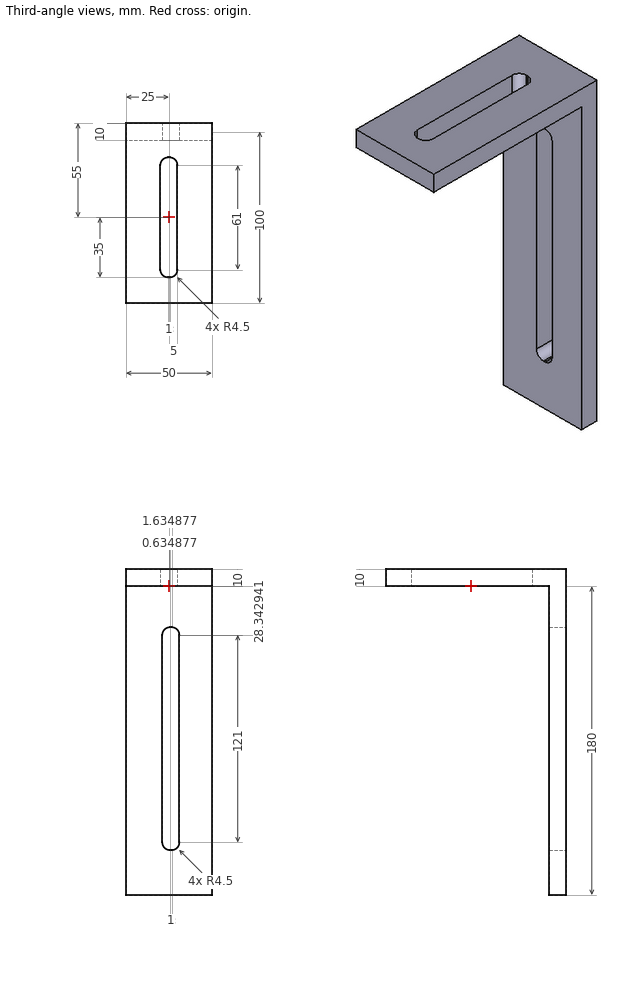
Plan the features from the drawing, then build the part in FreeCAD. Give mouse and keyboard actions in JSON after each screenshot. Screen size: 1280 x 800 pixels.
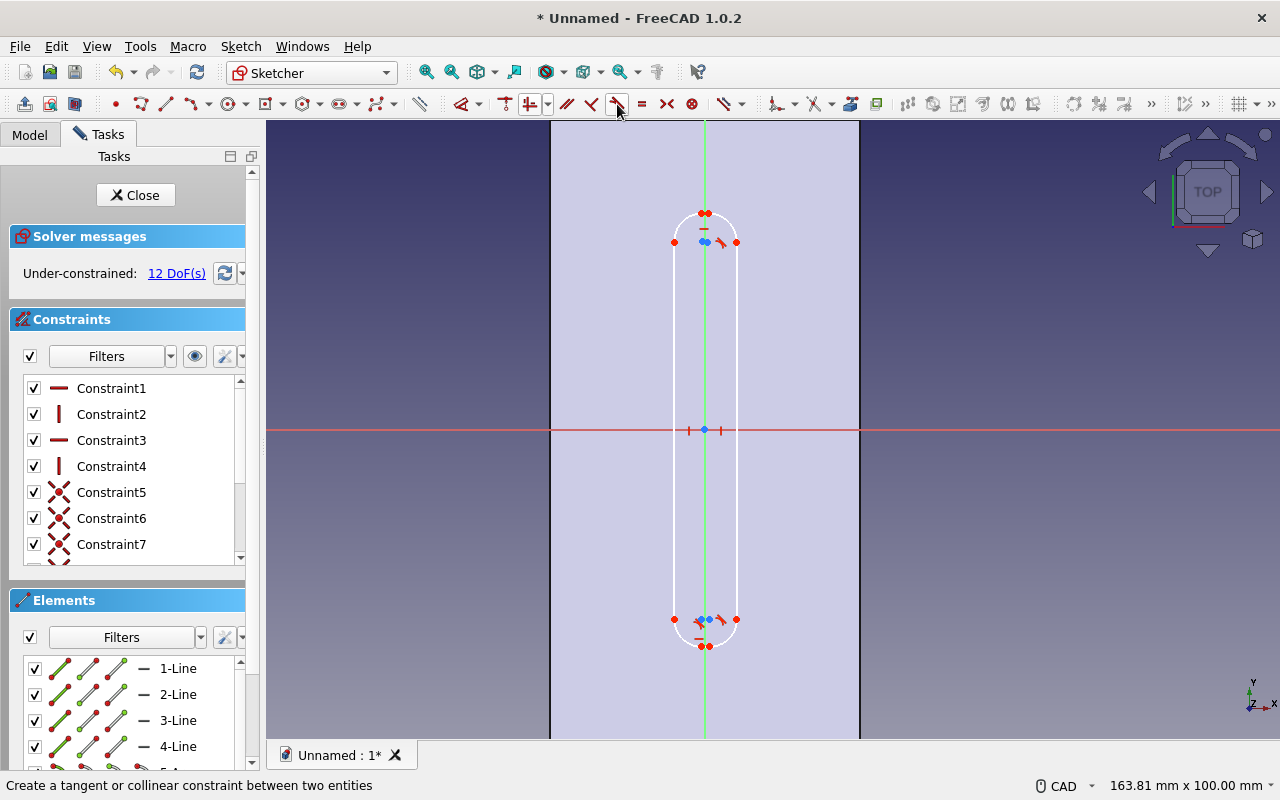
{"action": "scroll", "coordinate": [705, 213], "scroll_direction": "up", "scroll_amount": 8}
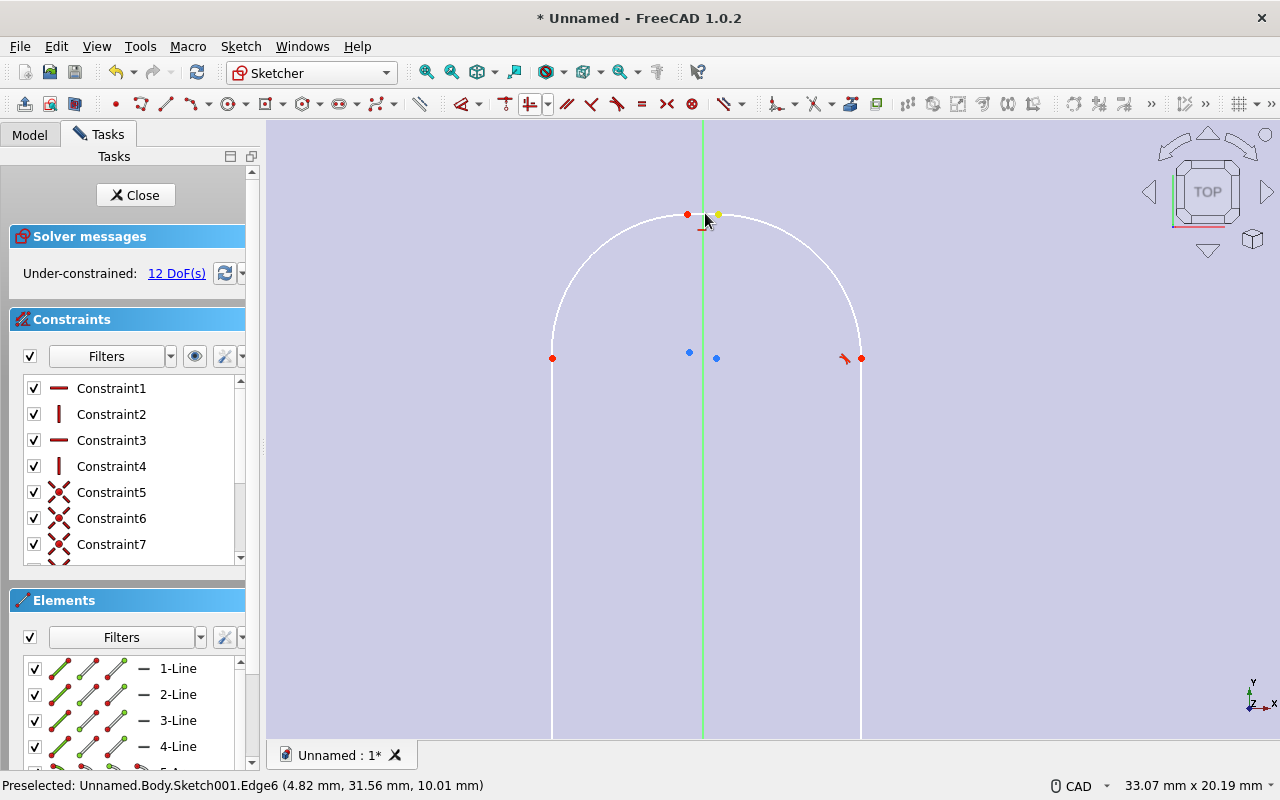
{"action": "left_click", "coordinate": [703, 214]}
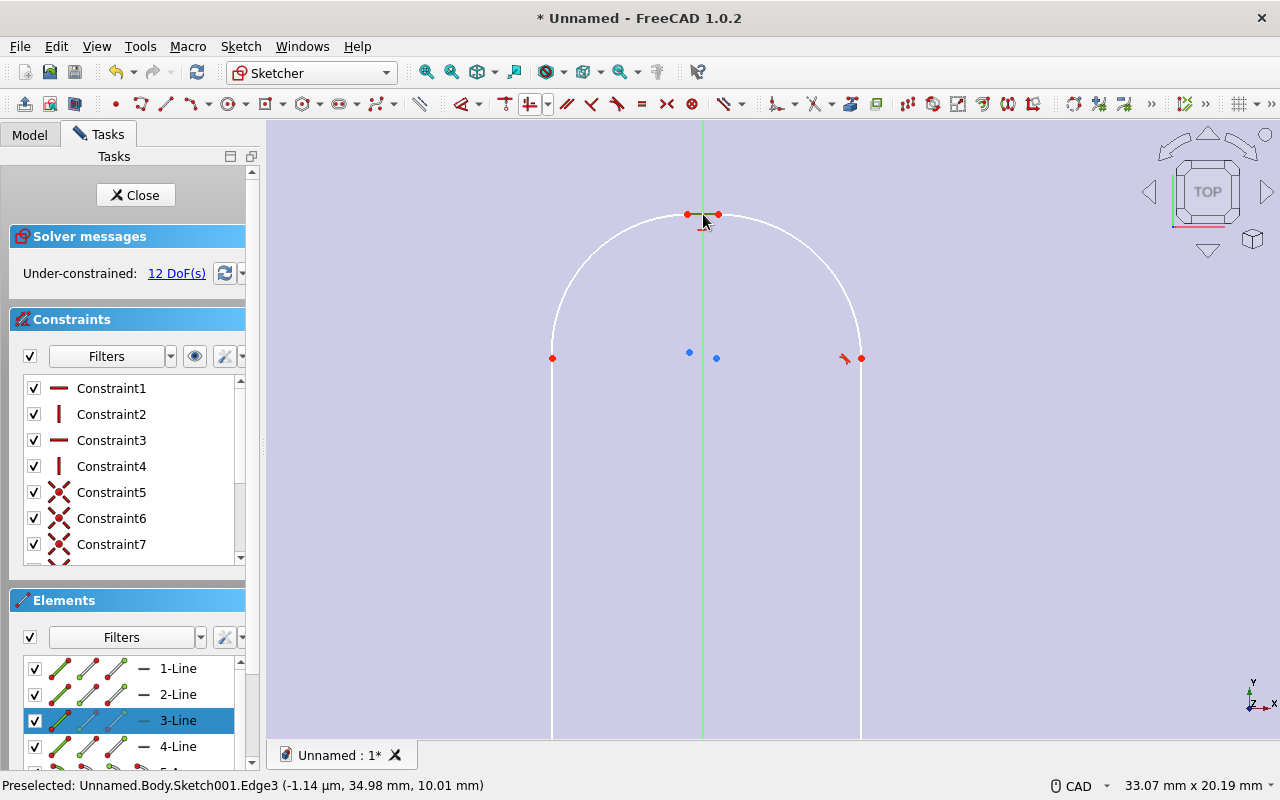
{"action": "scroll", "coordinate": [705, 213], "scroll_direction": "down", "scroll_amount": 8}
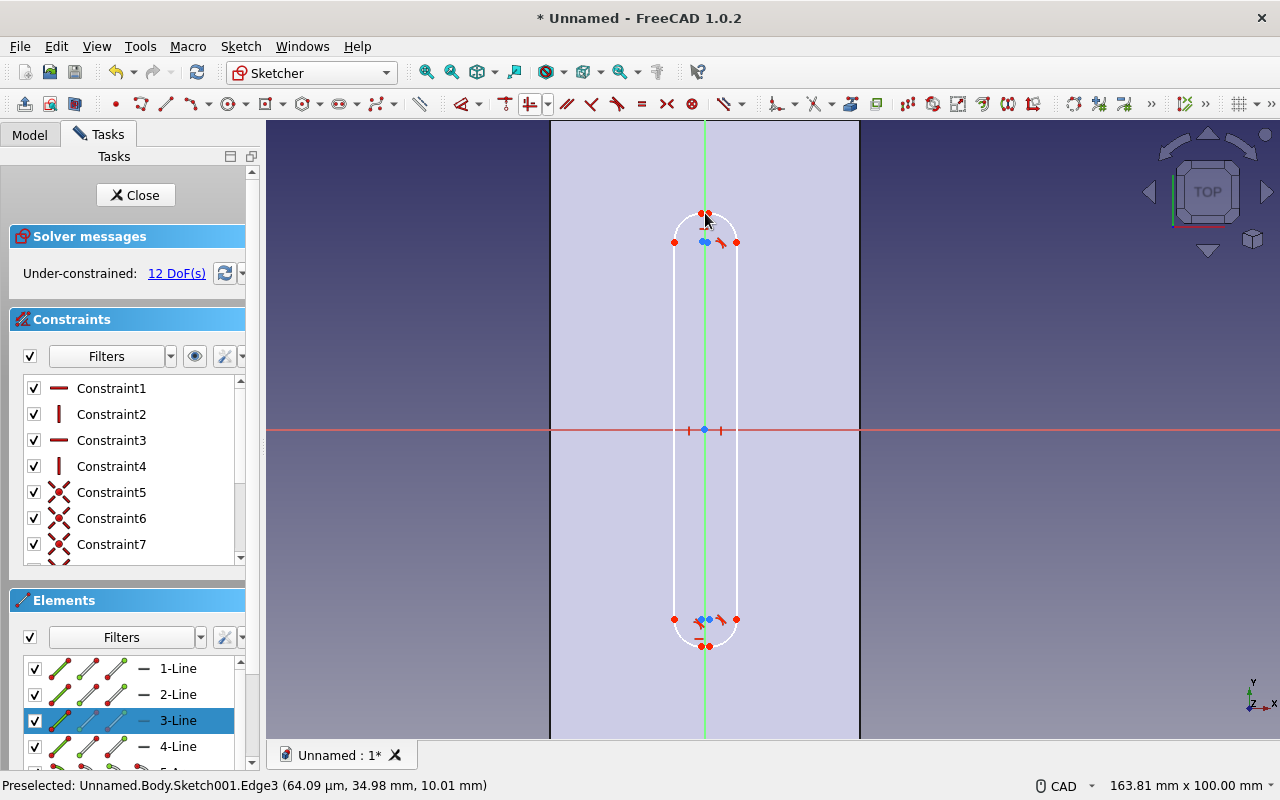
{"action": "left_click", "coordinate": [734, 229]}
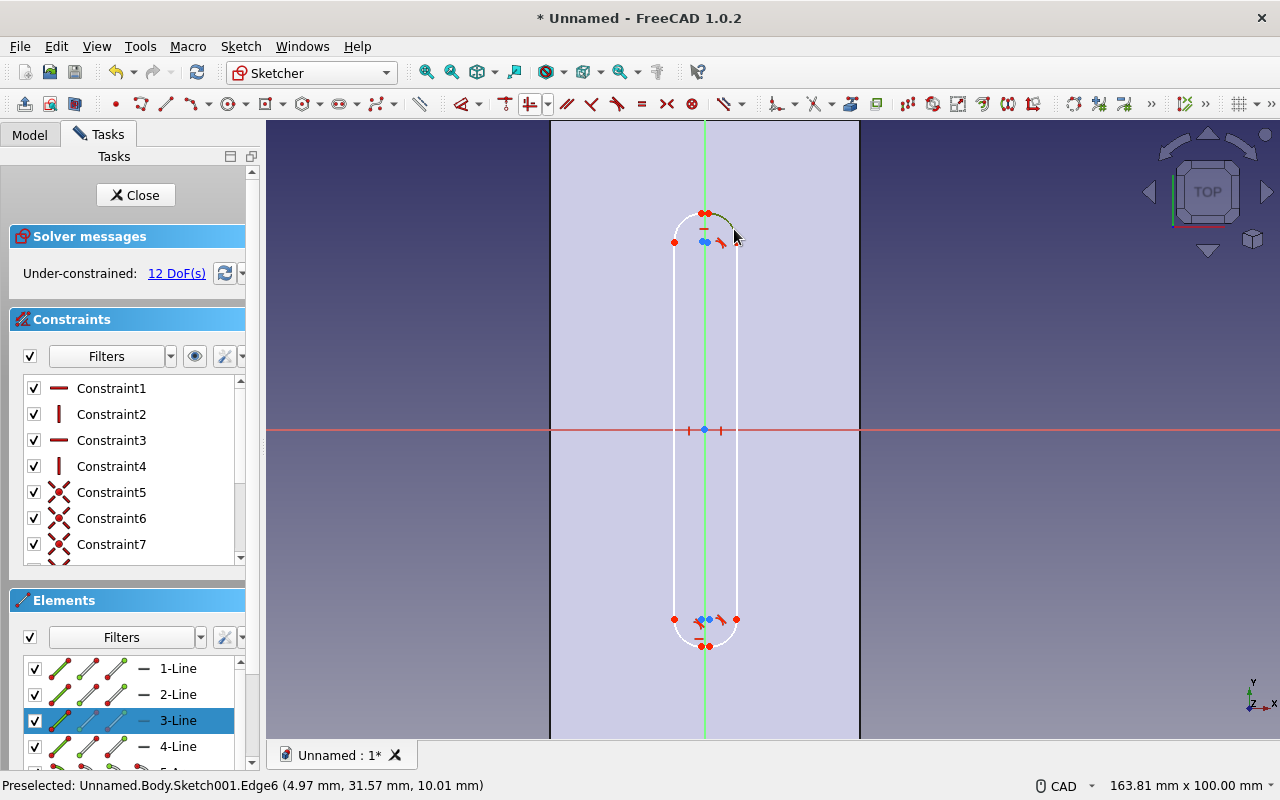
{"action": "left_click", "coordinate": [617, 104]}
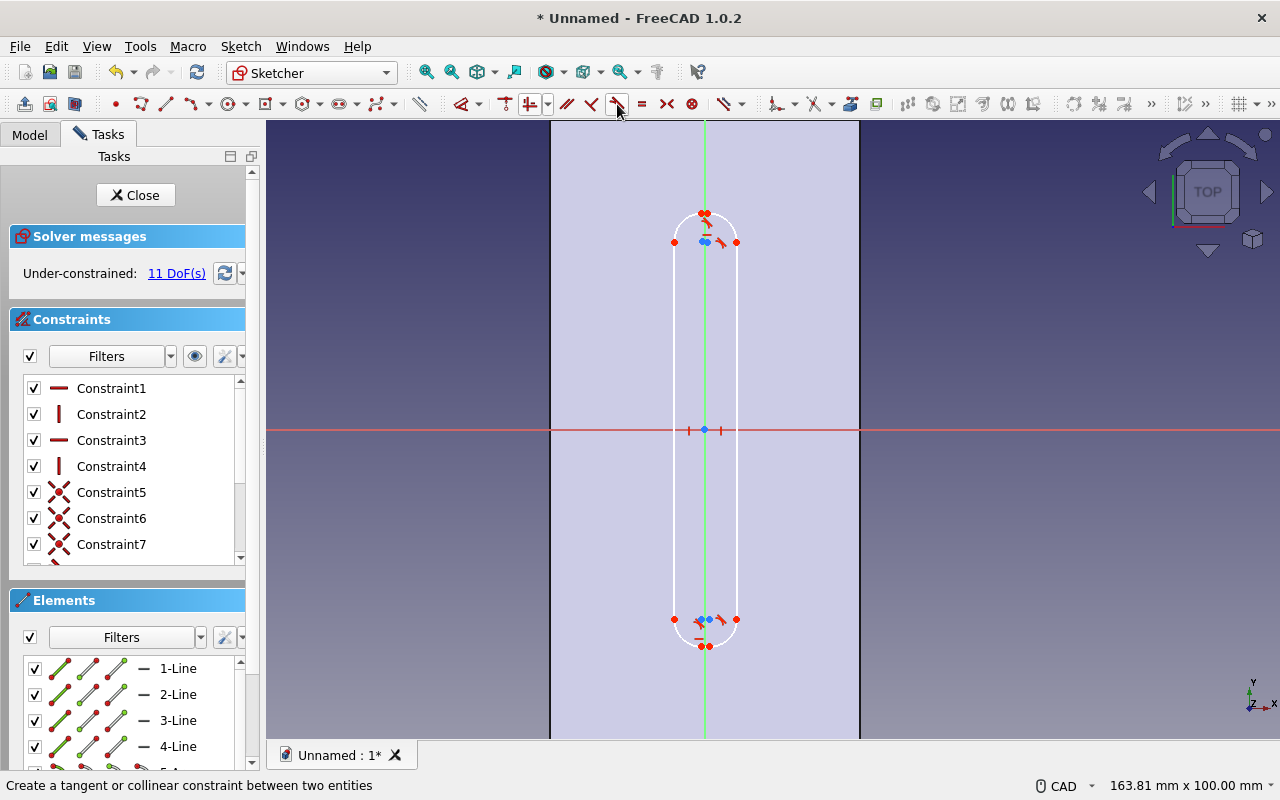
{"action": "scroll", "coordinate": [705, 213], "scroll_direction": "up", "scroll_amount": 8}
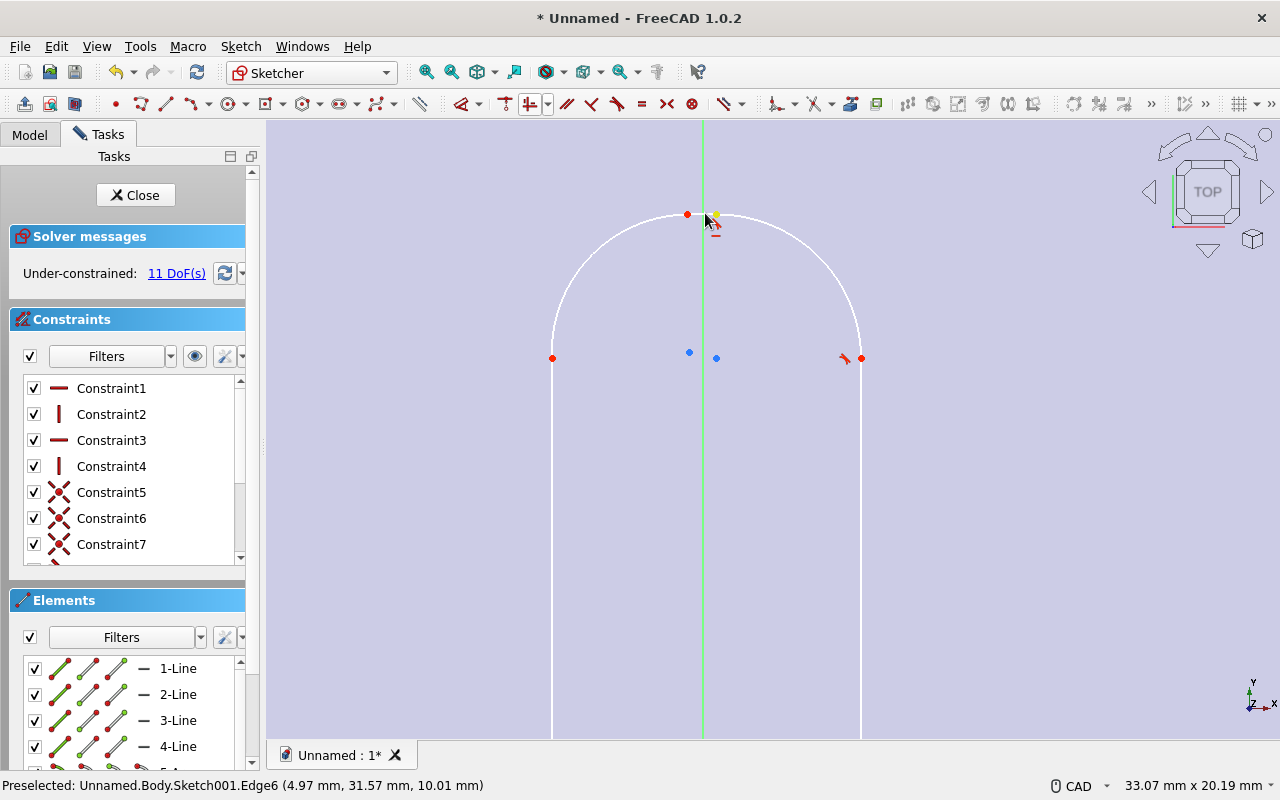
{"action": "left_click", "coordinate": [702, 214]}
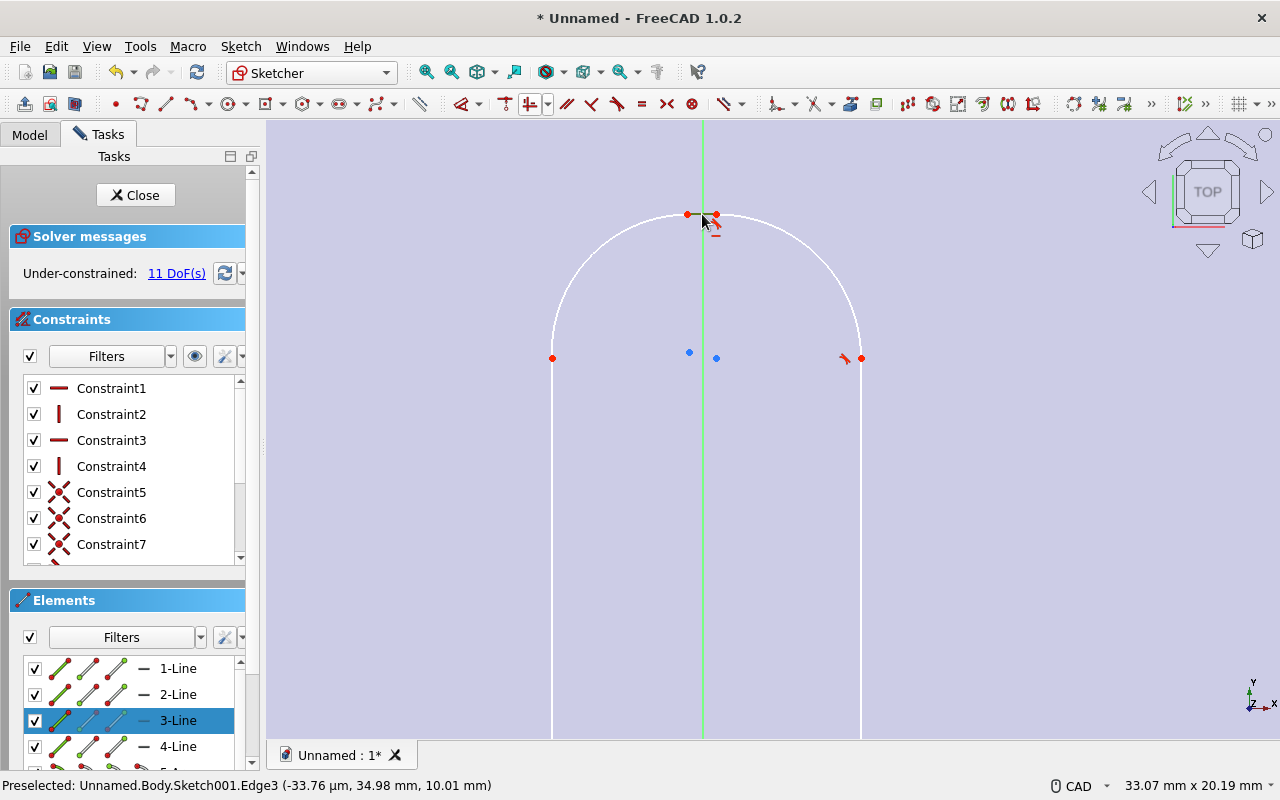
{"action": "scroll", "coordinate": [705, 213], "scroll_direction": "down", "scroll_amount": 8}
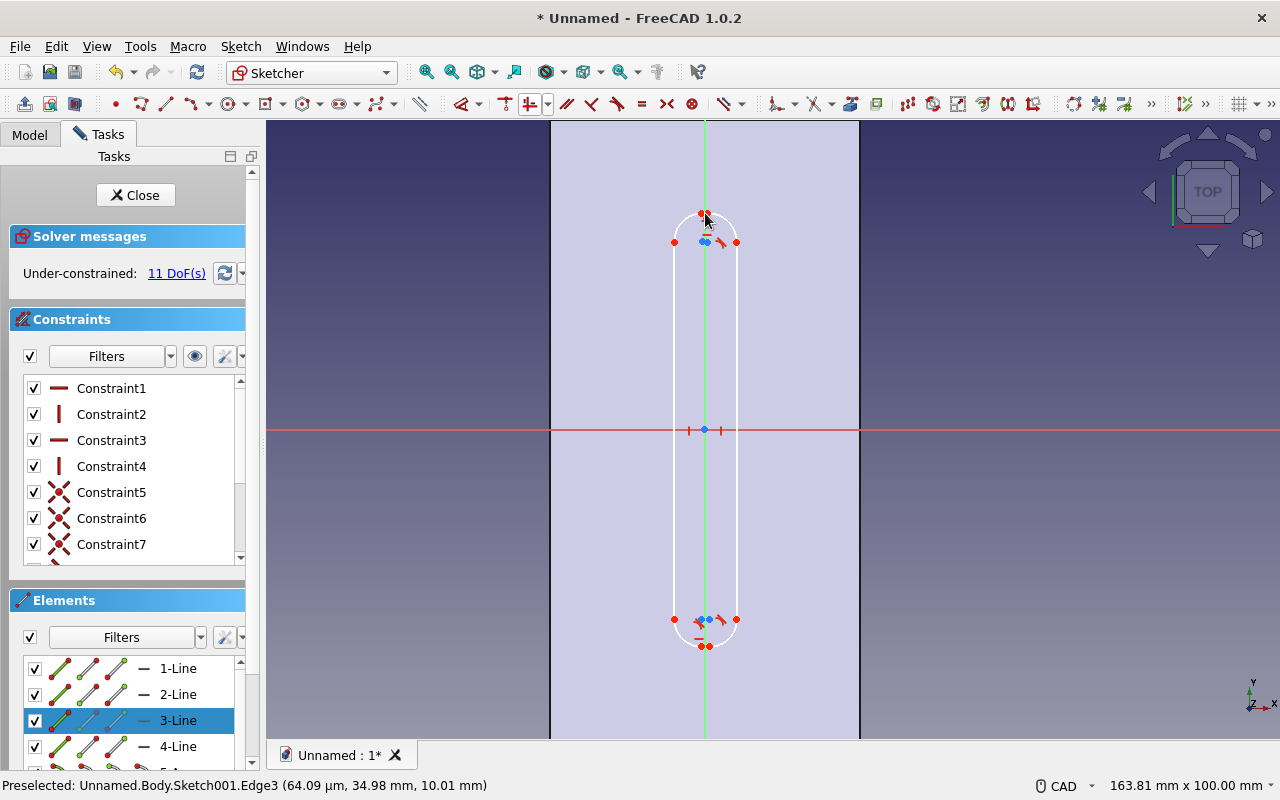
{"action": "left_click", "coordinate": [689, 217]}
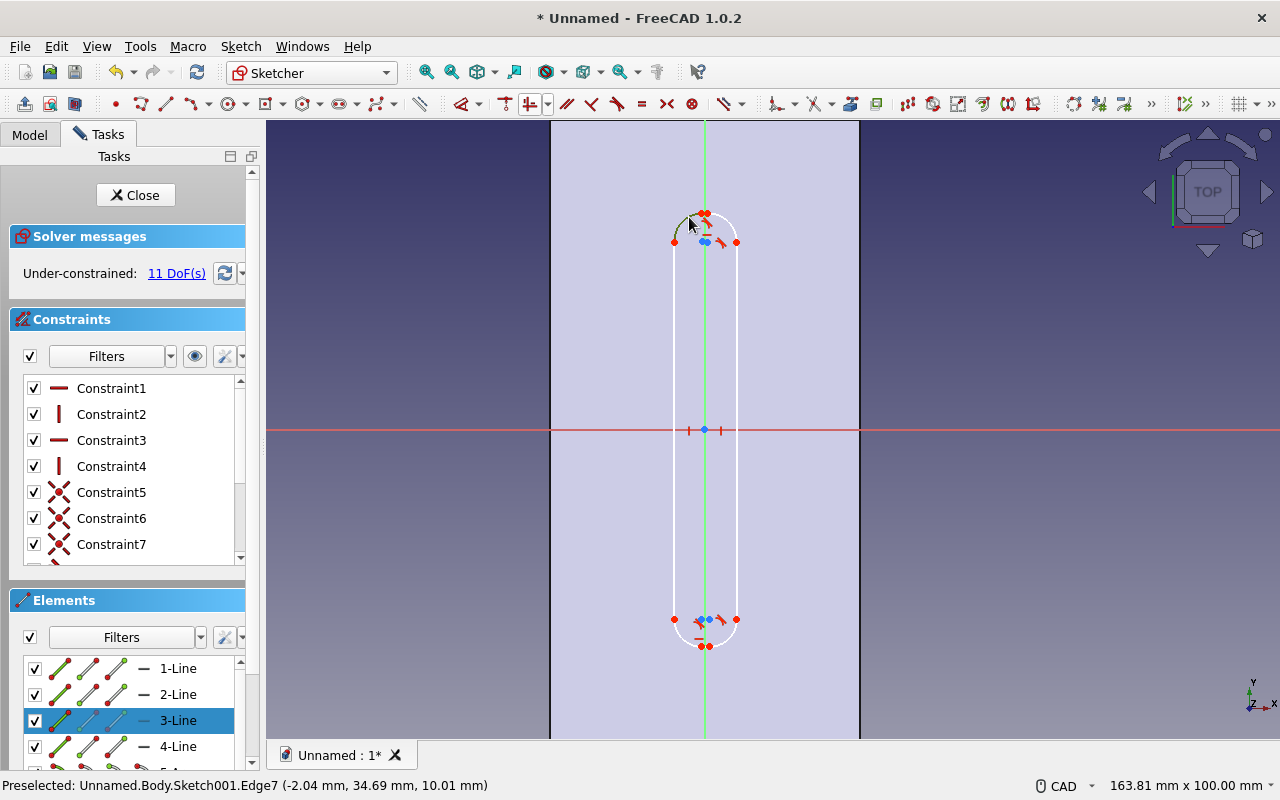
{"action": "left_click", "coordinate": [617, 104]}